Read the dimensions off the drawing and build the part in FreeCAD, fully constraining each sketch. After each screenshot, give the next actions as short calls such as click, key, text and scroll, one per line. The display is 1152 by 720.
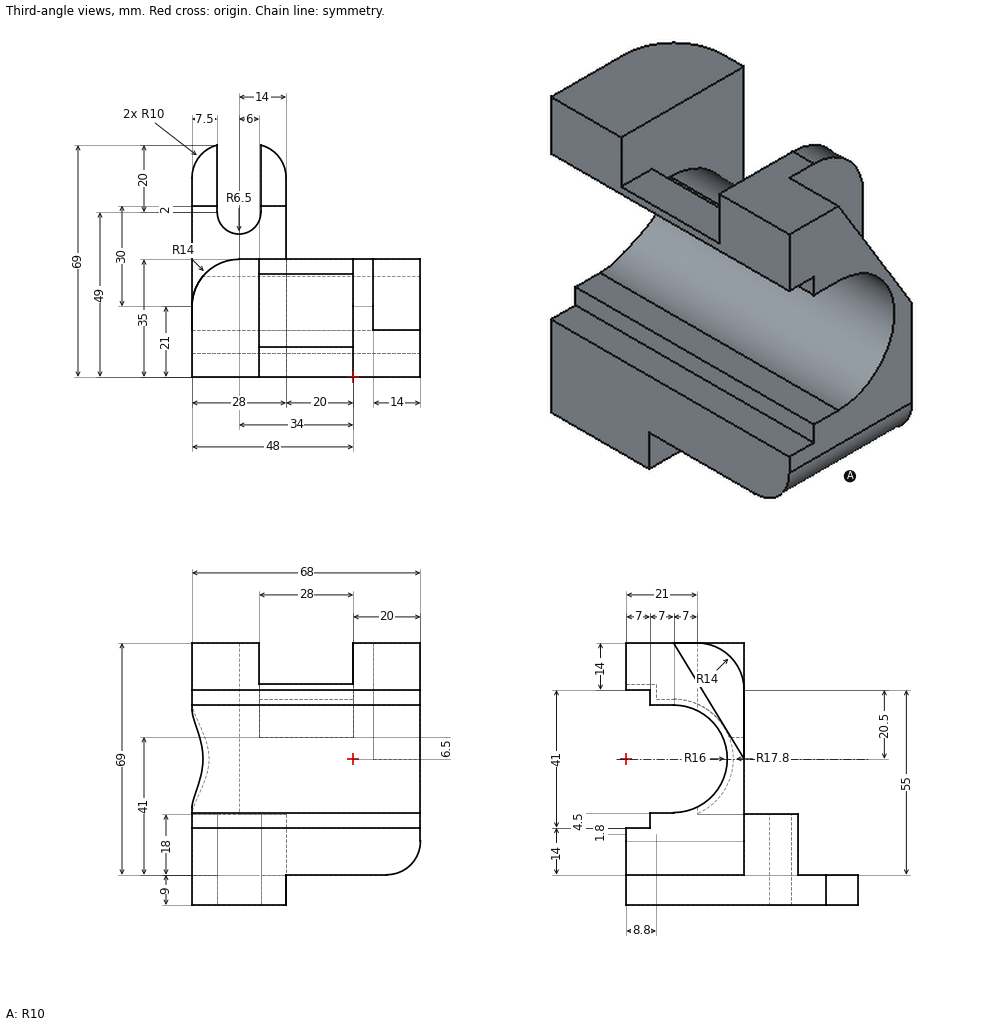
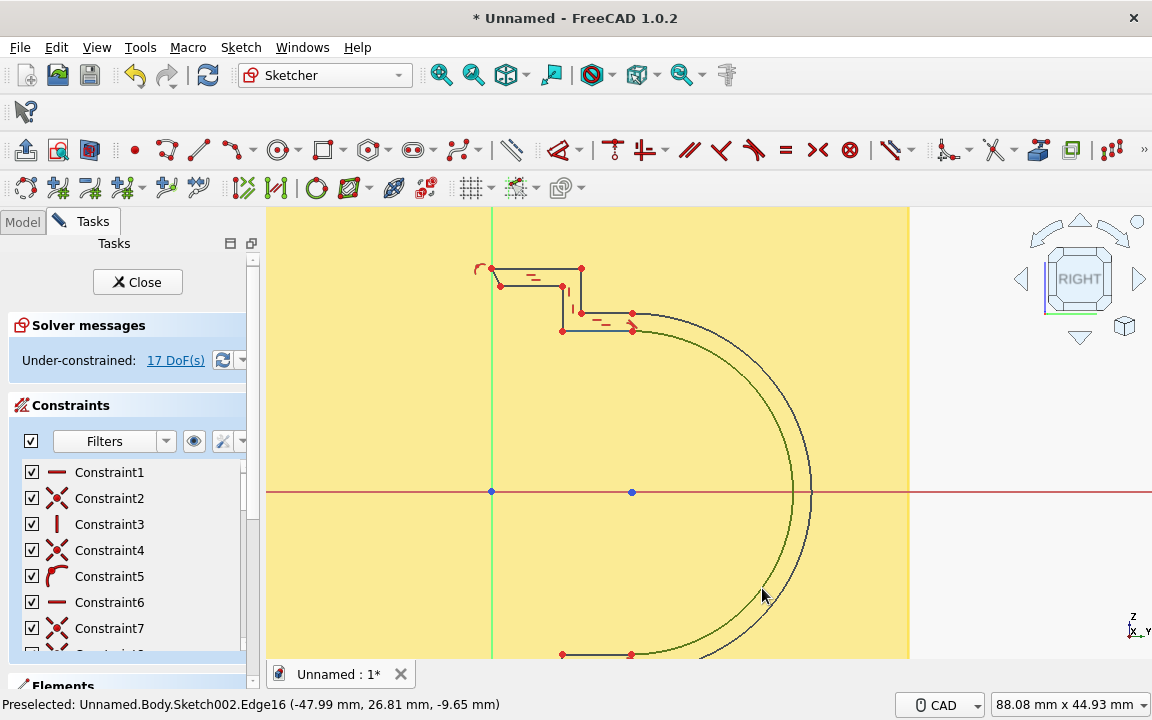
click(754, 150)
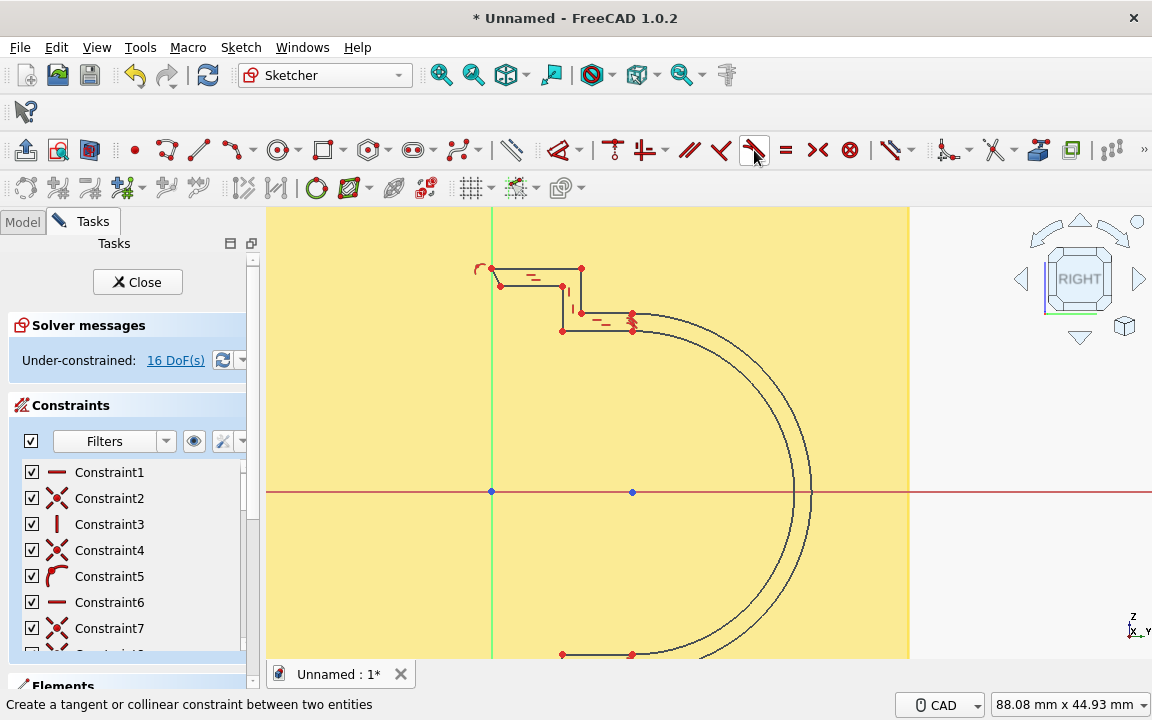
scroll(617, 314, down, 2)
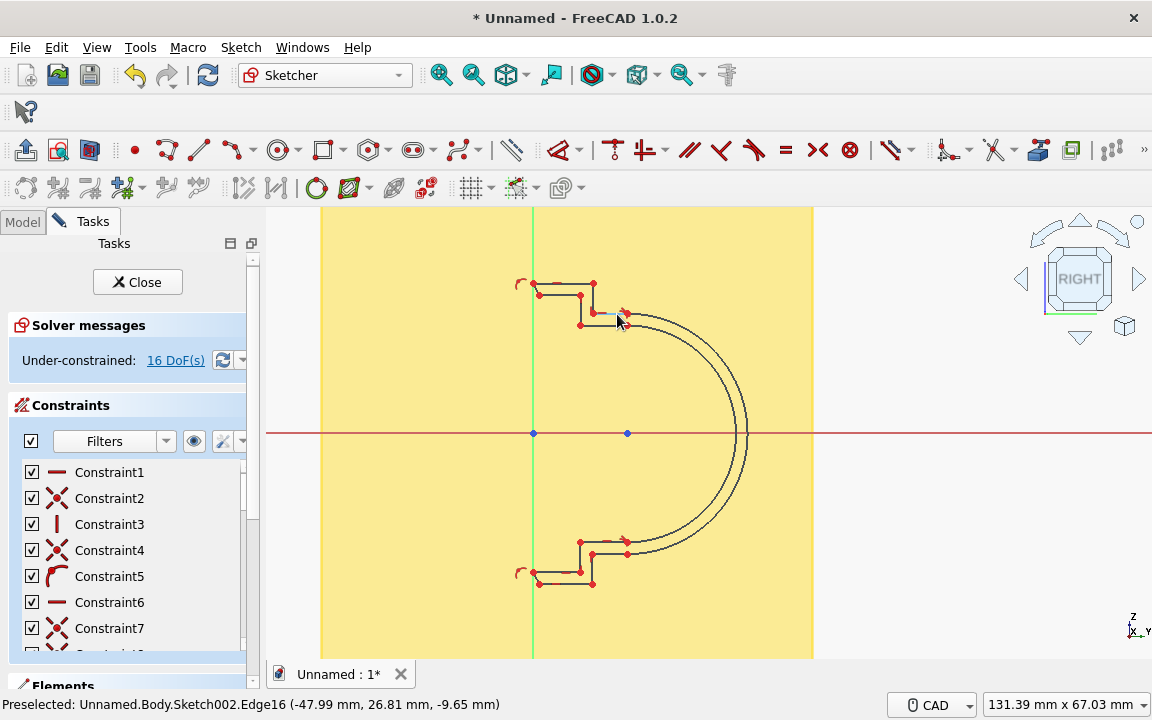
scroll(536, 577, up, 6)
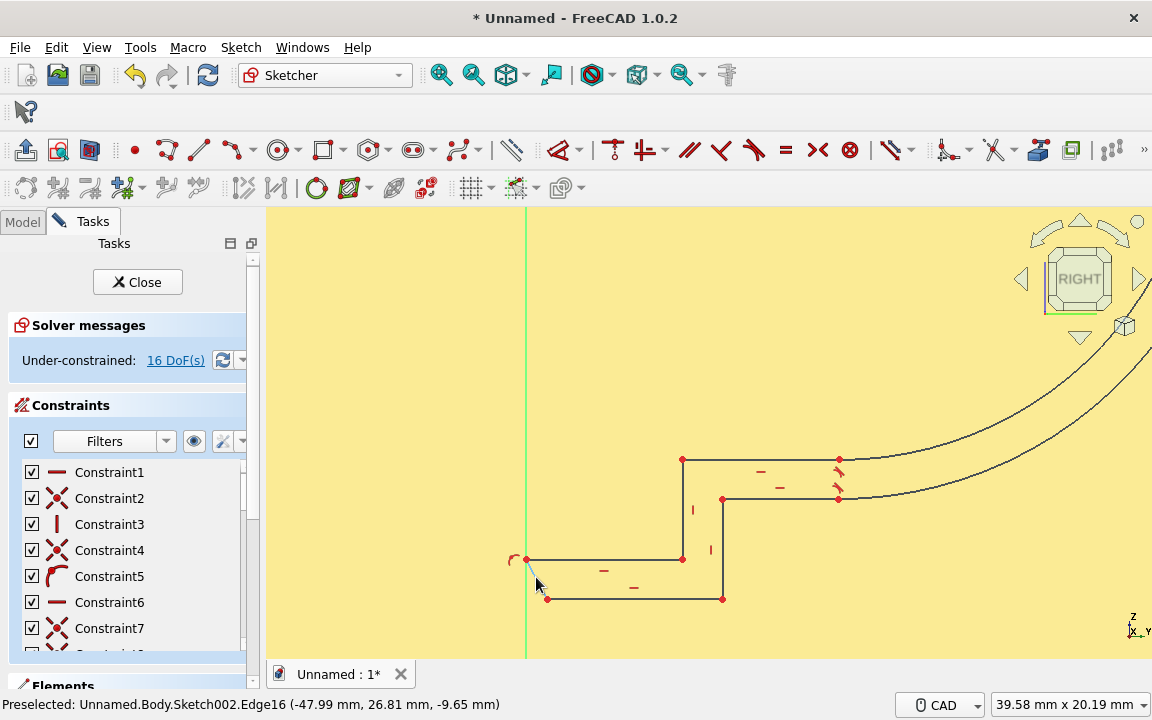
click(535, 575)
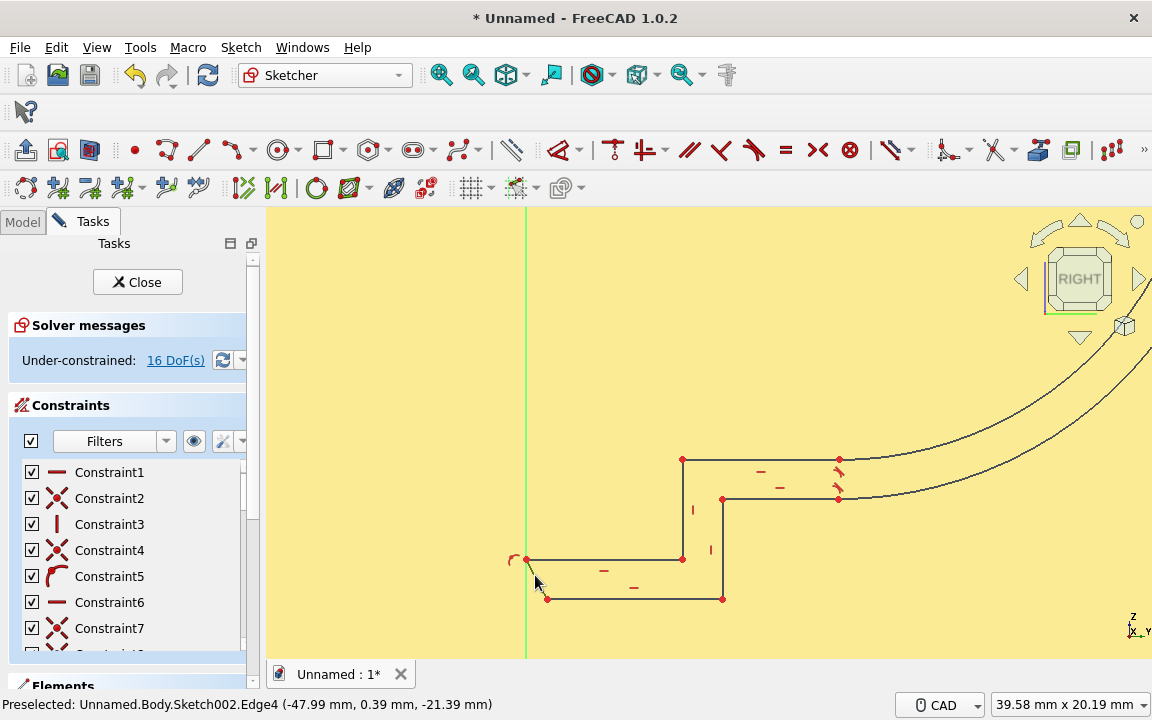
key(v)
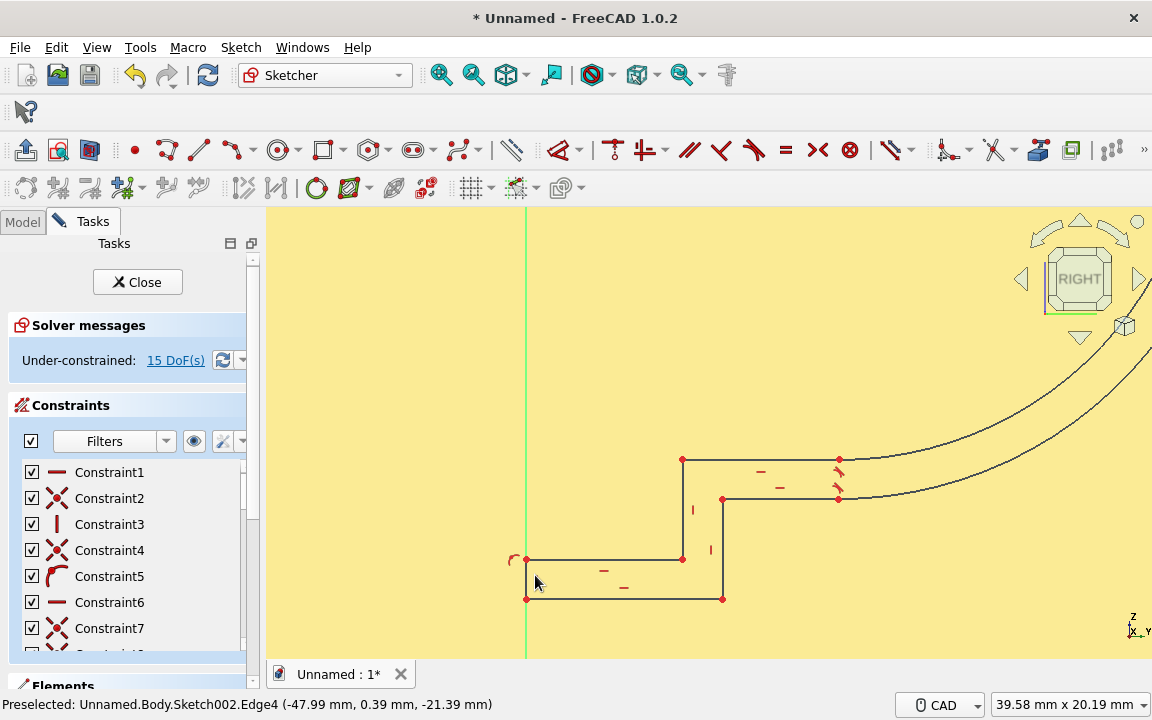
scroll(536, 578, down, 6)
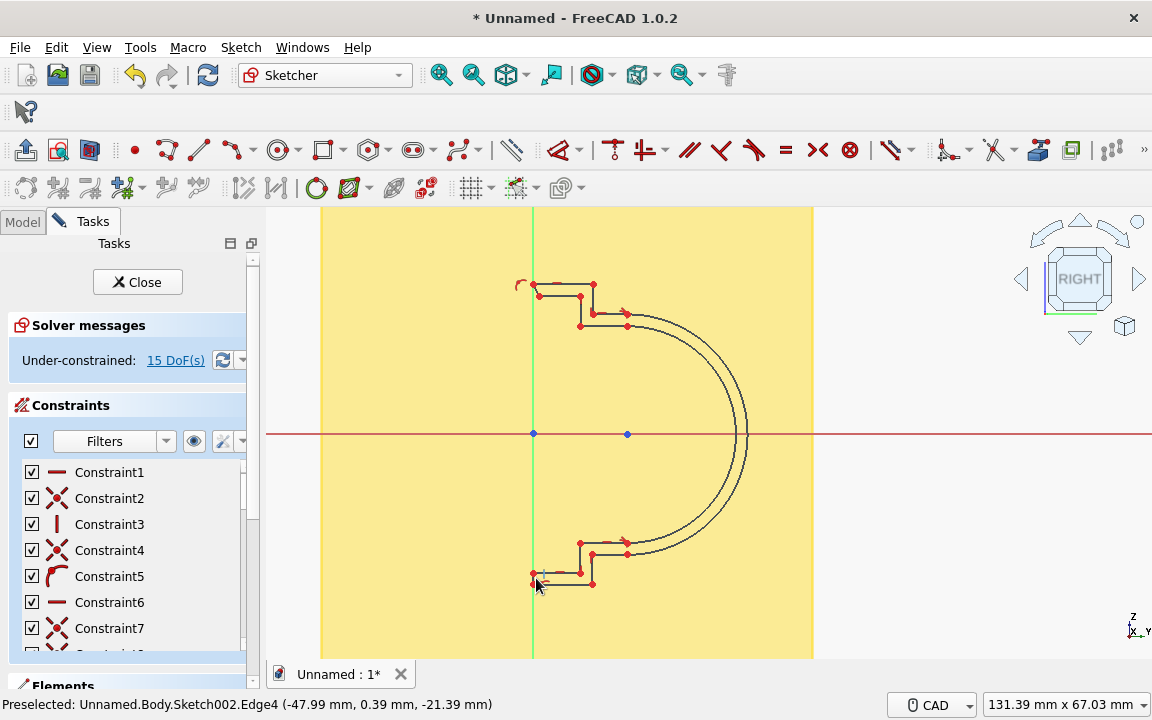
scroll(537, 293, up, 7)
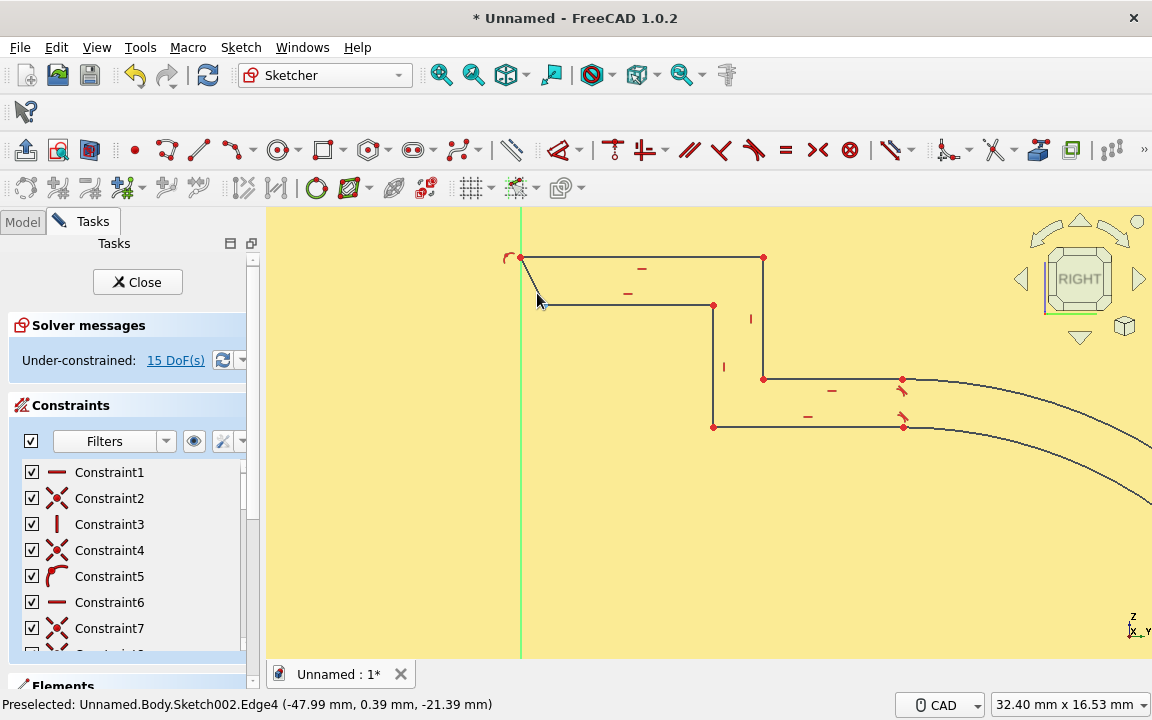
click(538, 291)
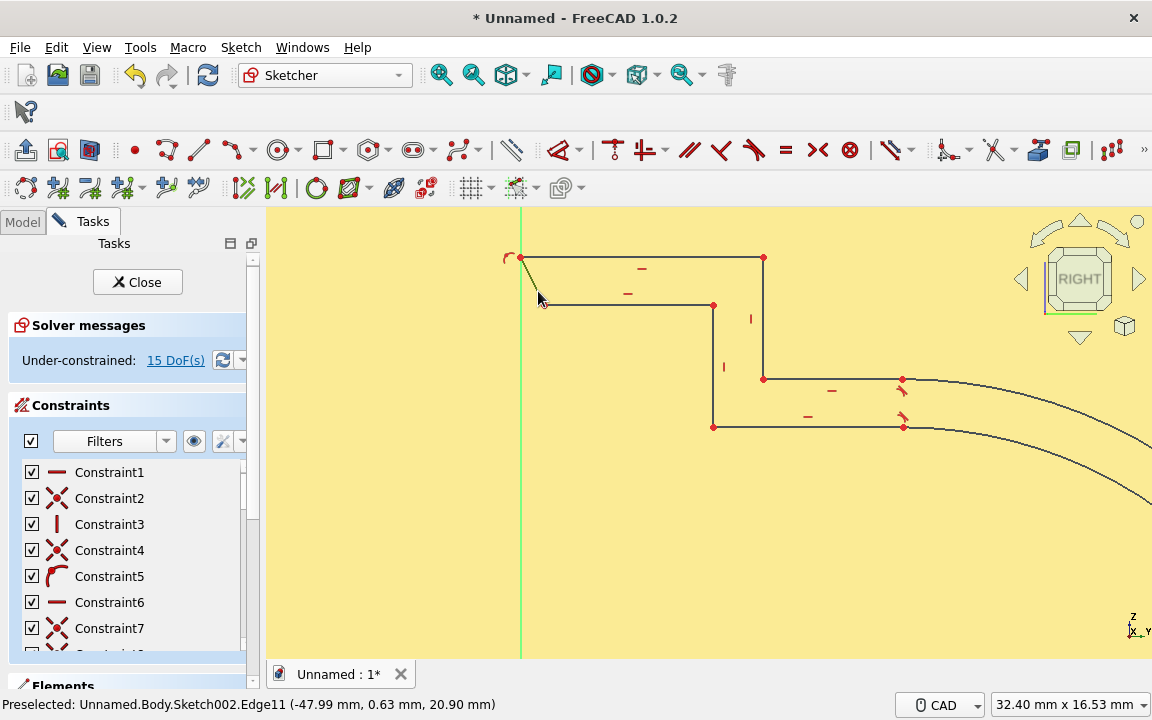
key(v)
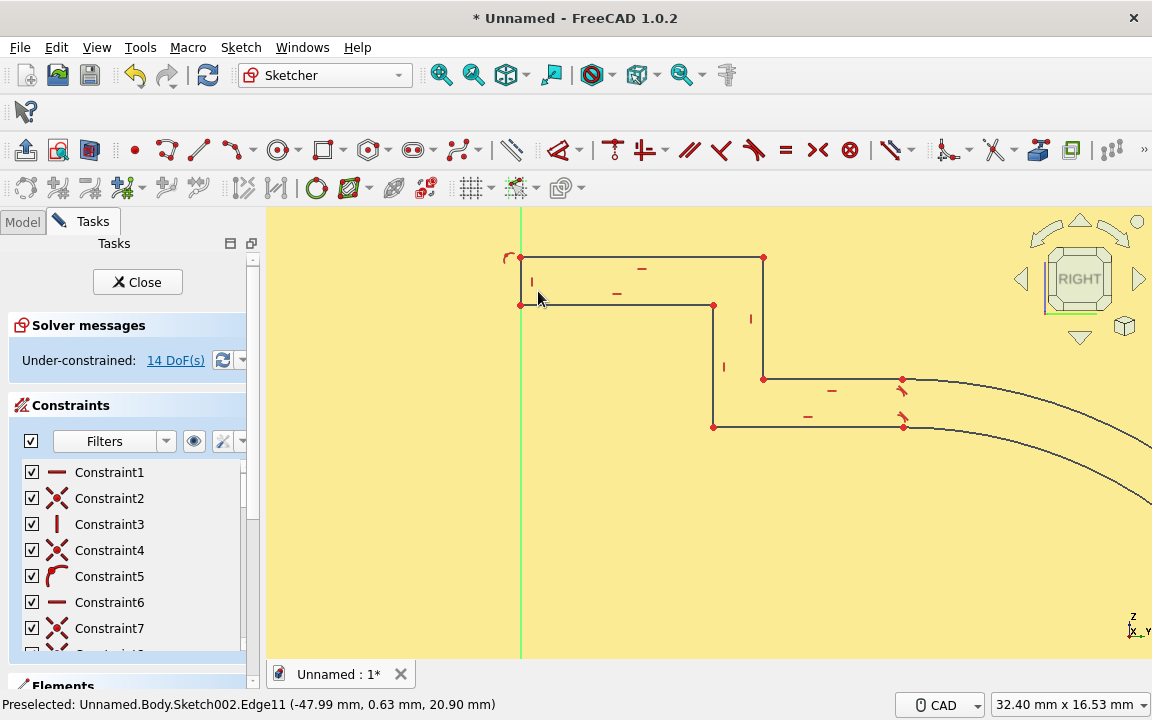
scroll(537, 292, down, 7)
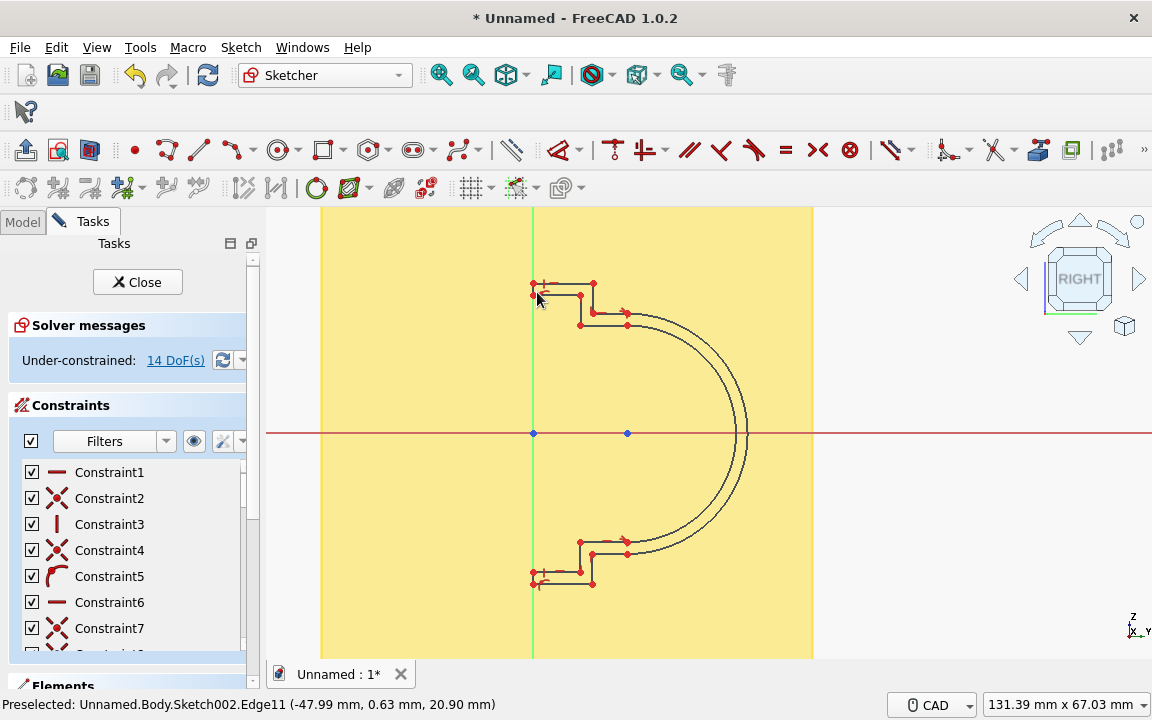
click(725, 504)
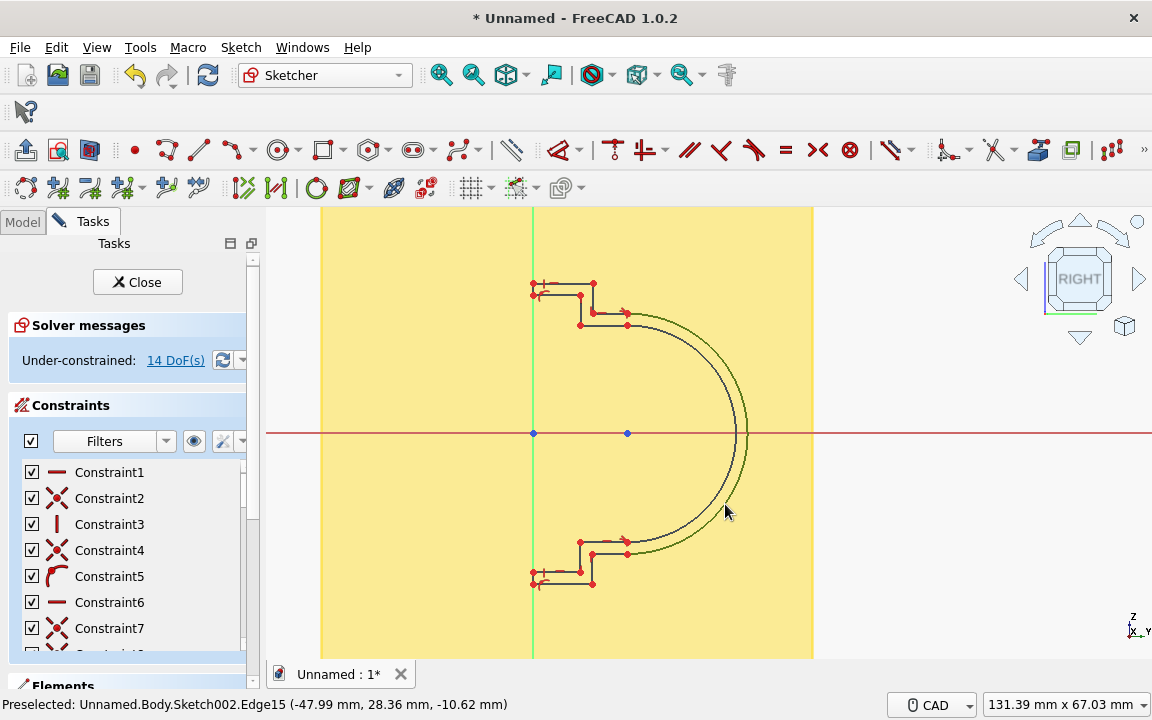
click(715, 498)